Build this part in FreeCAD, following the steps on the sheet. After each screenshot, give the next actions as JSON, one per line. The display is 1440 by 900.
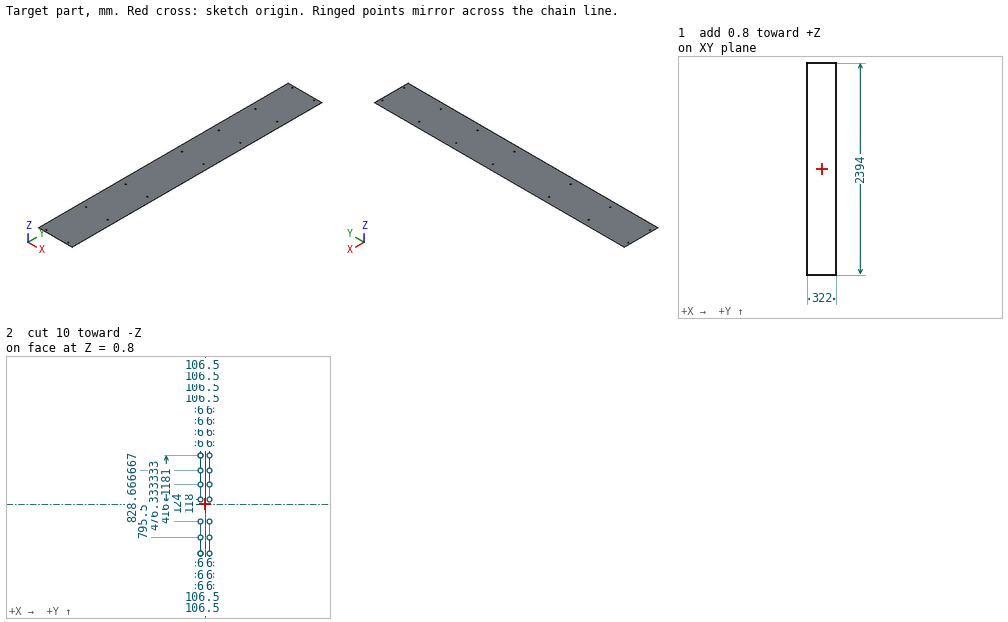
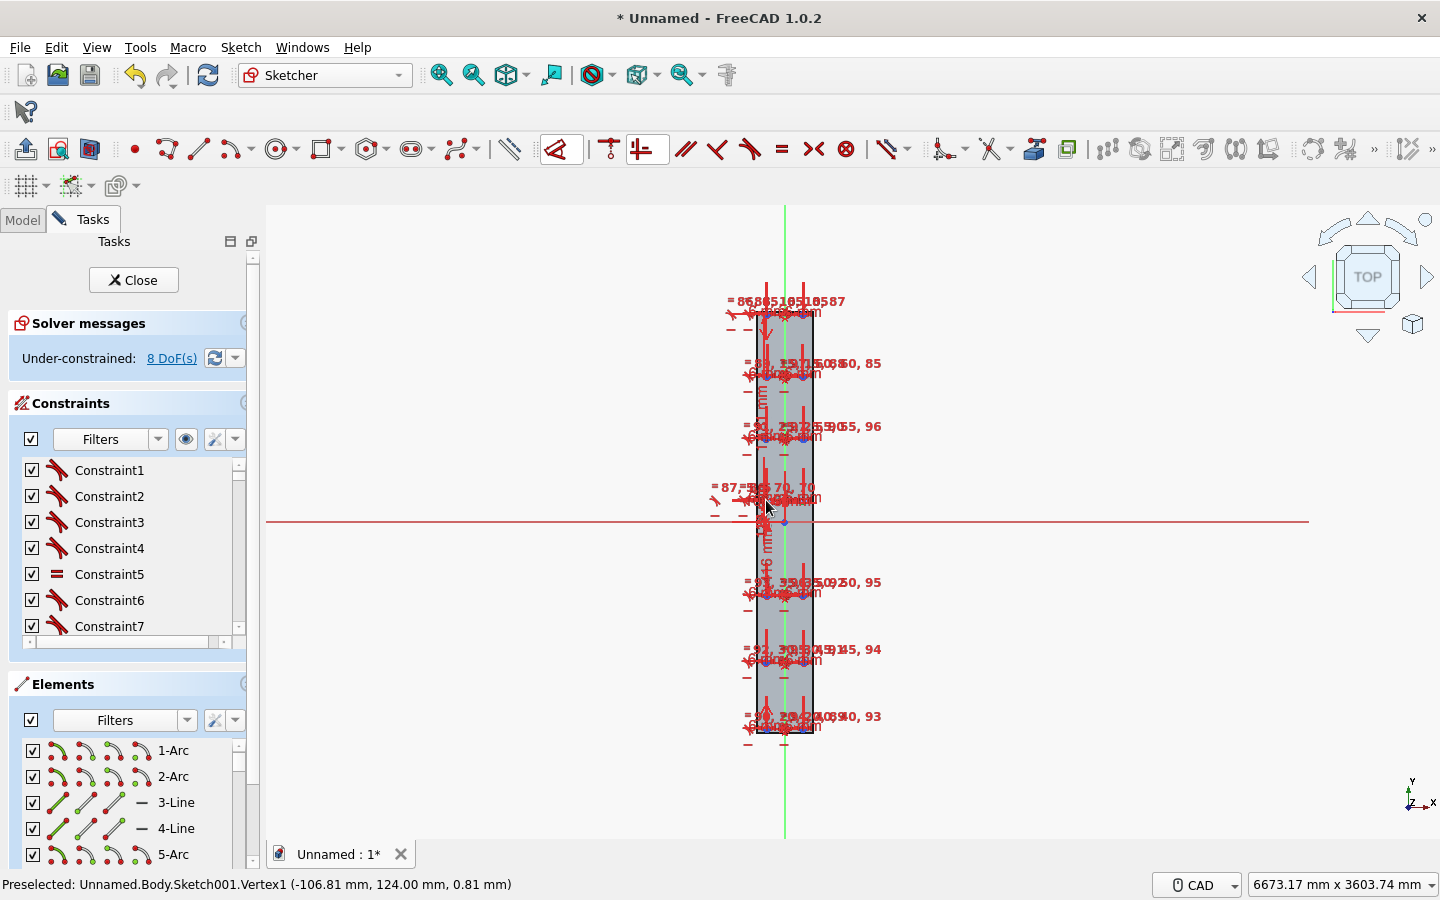
{"action": "scroll", "coordinate": [766, 314], "scroll_direction": "up", "scroll_amount": 14}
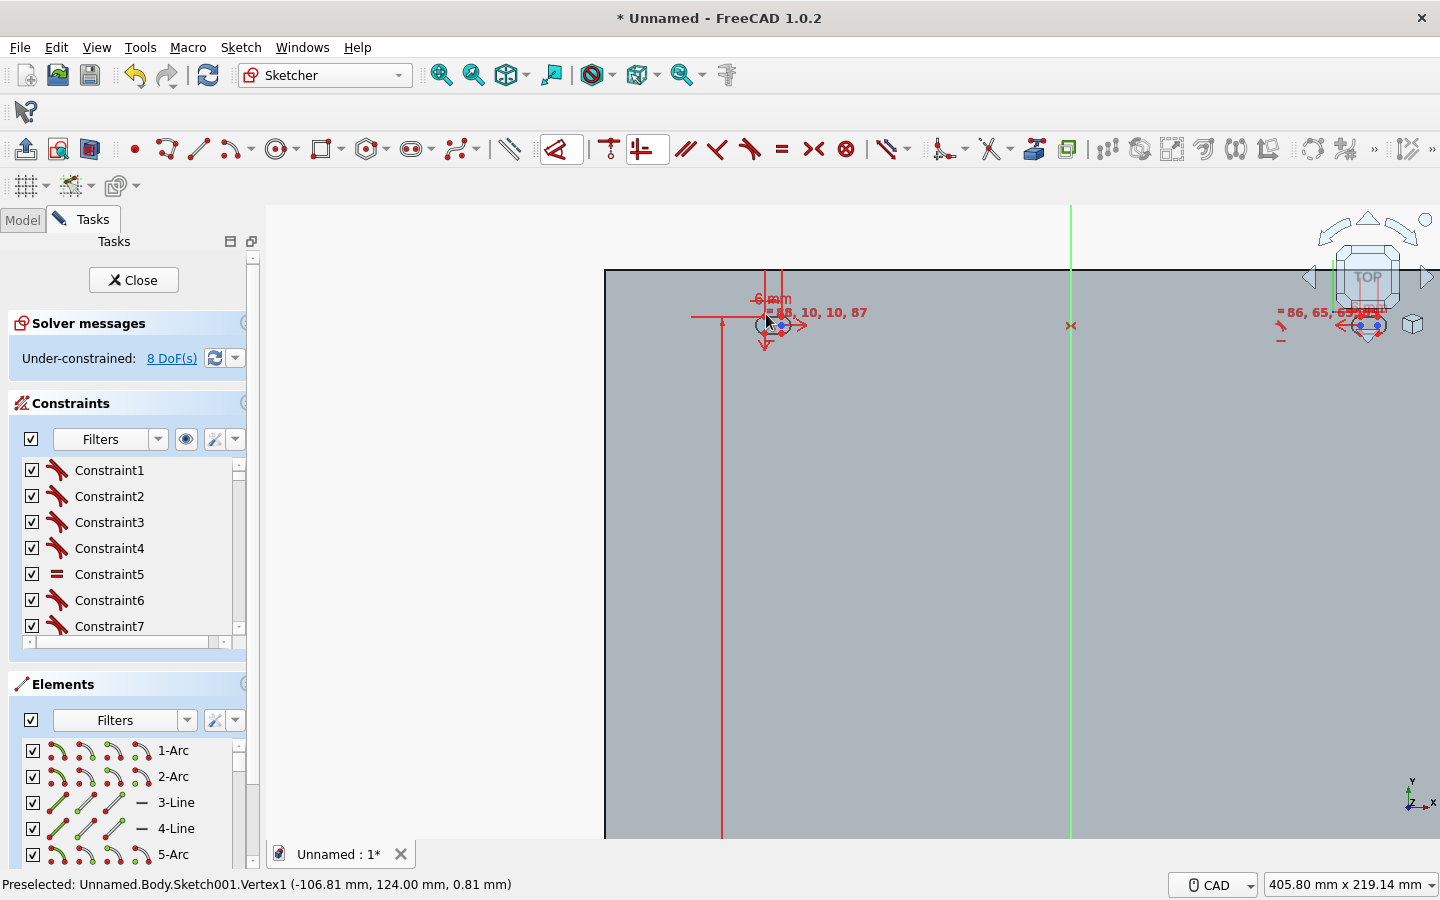
{"action": "left_click", "coordinate": [765, 317]}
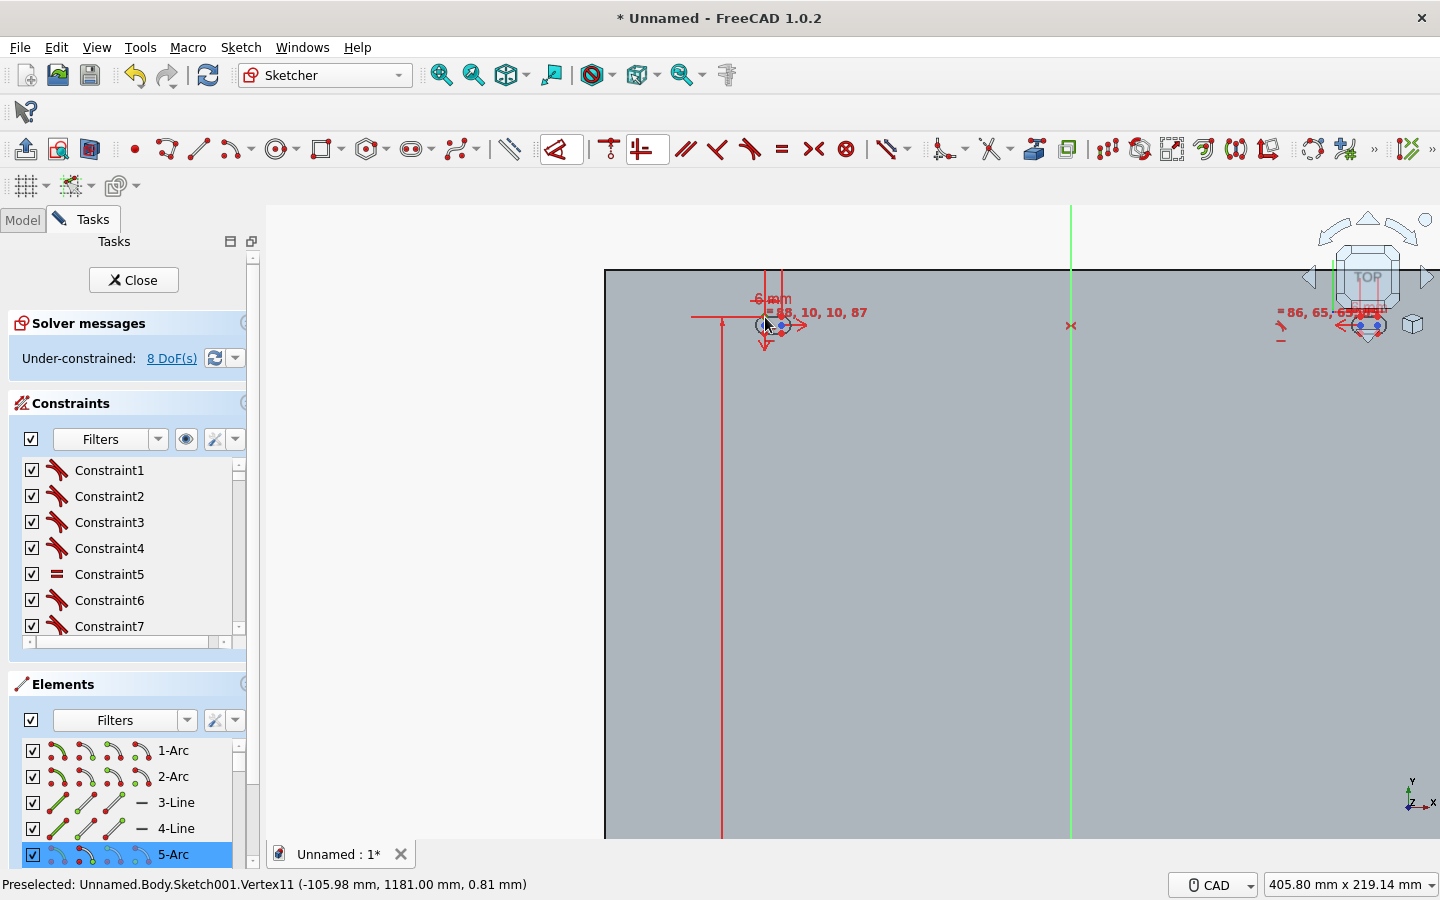
{"action": "key", "text": "l"}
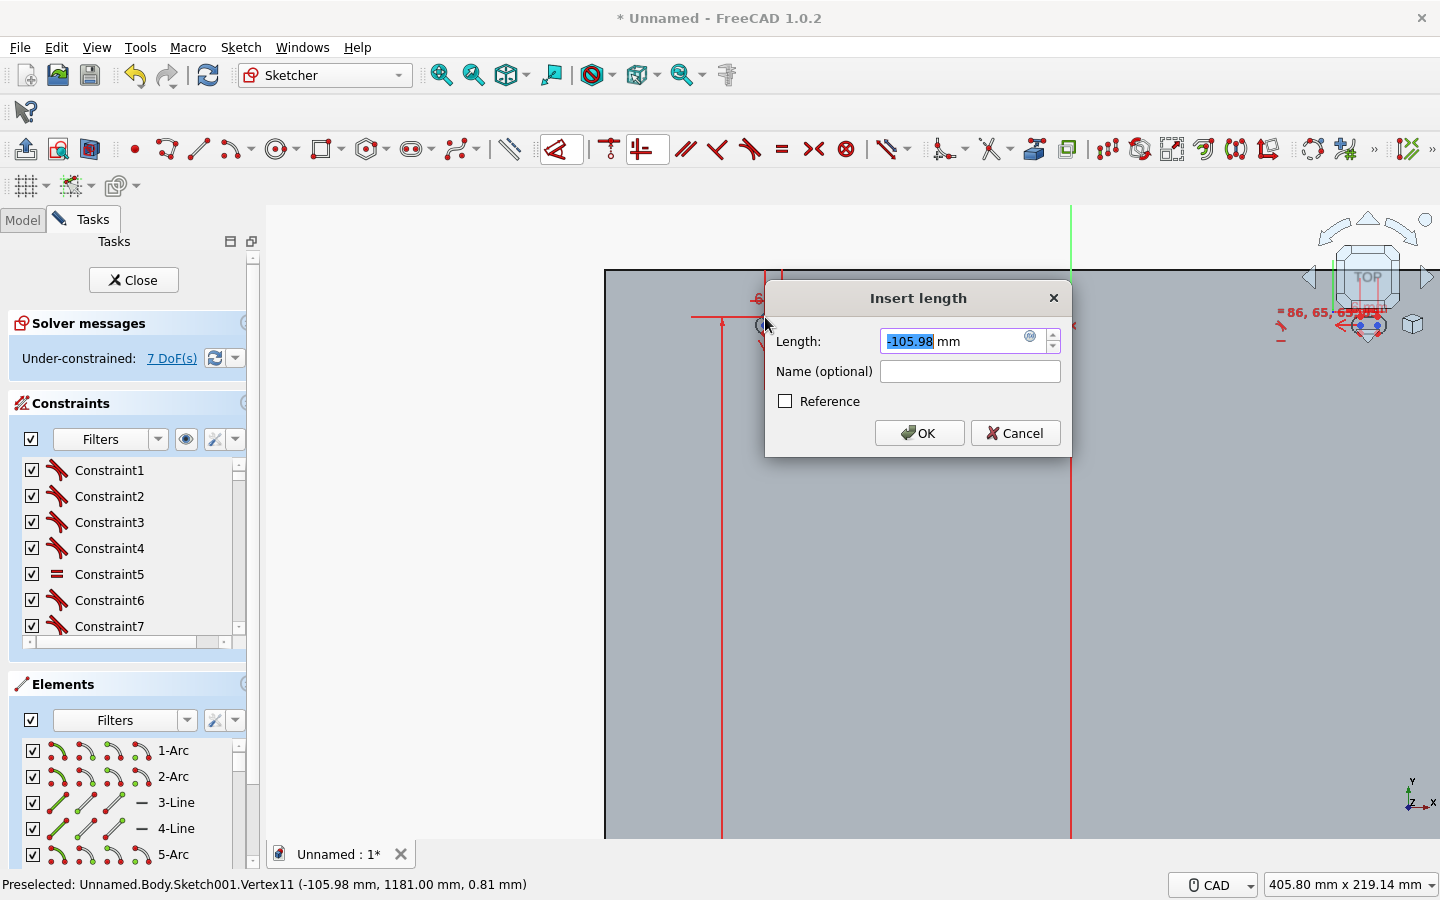
{"action": "type", "text": "-106.5"}
{"action": "key", "text": "Return"}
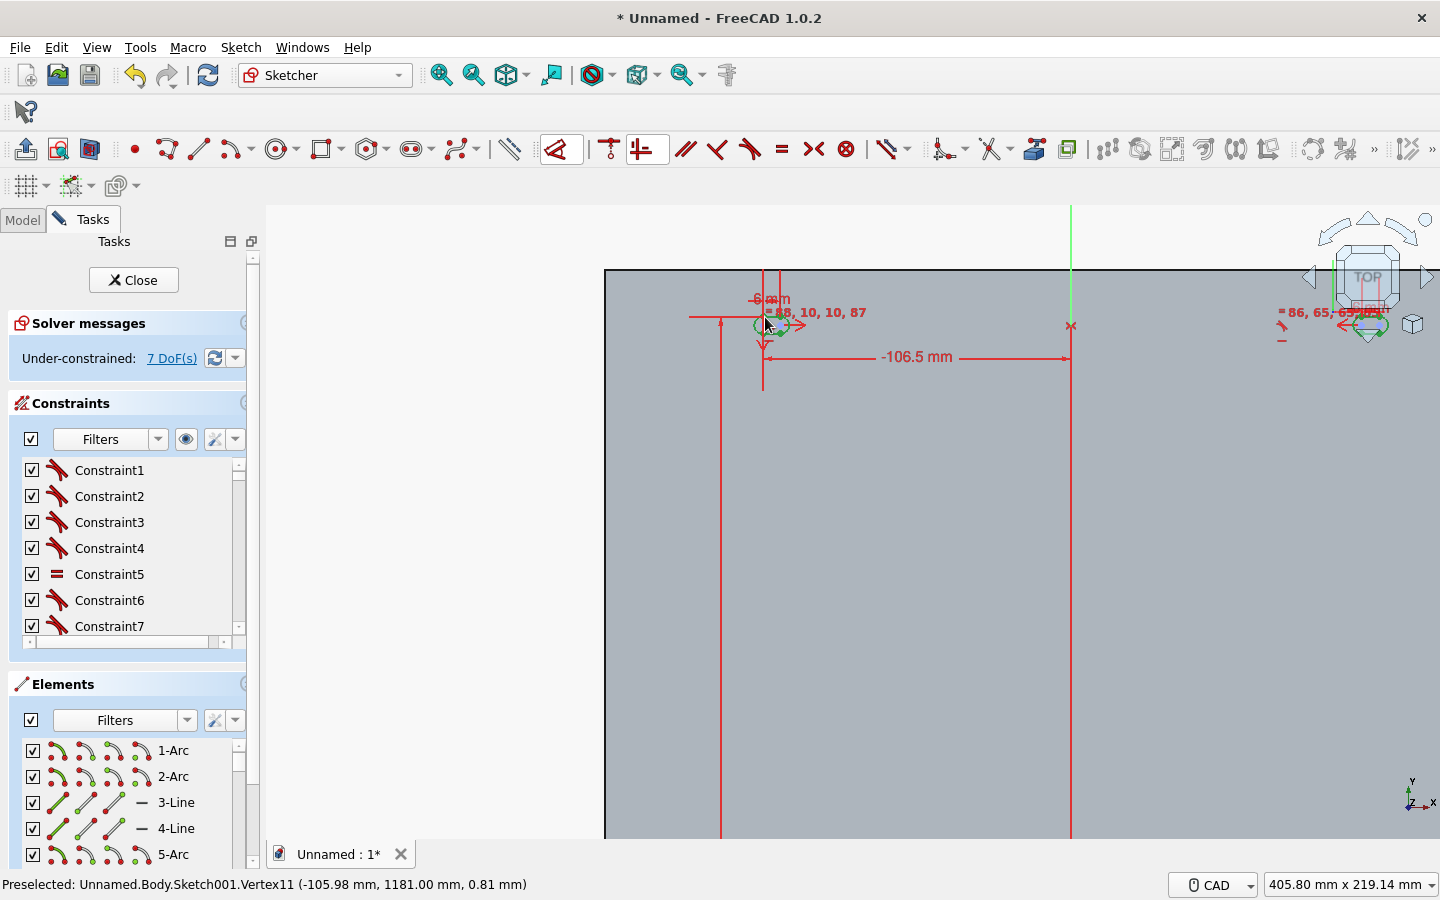
{"action": "scroll", "coordinate": [766, 314], "scroll_direction": "down", "scroll_amount": 14}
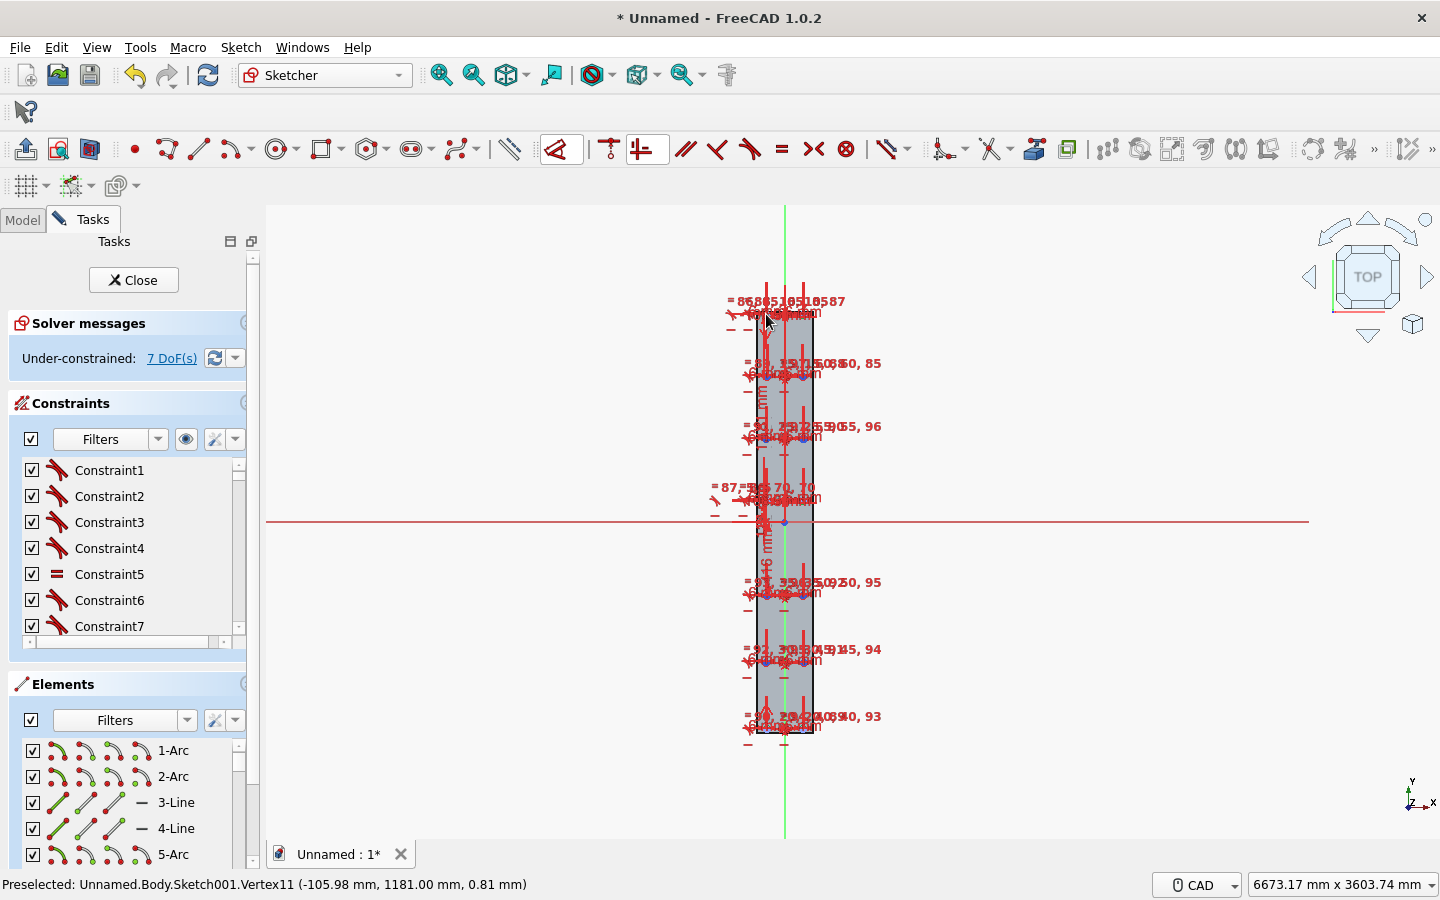
{"action": "scroll", "coordinate": [767, 376], "scroll_direction": "up", "scroll_amount": 14}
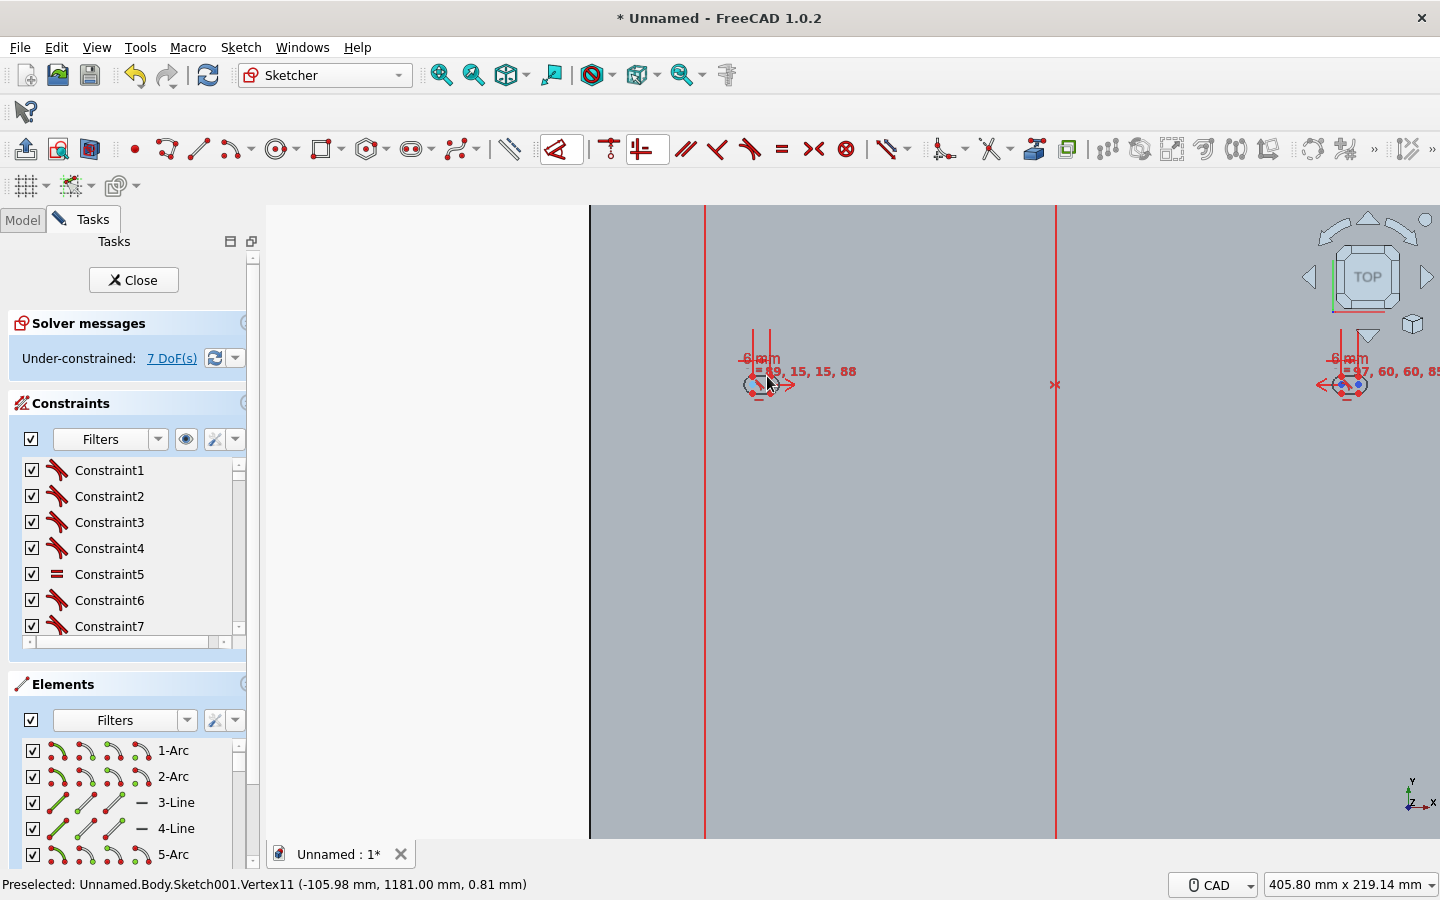
{"action": "left_click", "coordinate": [753, 376]}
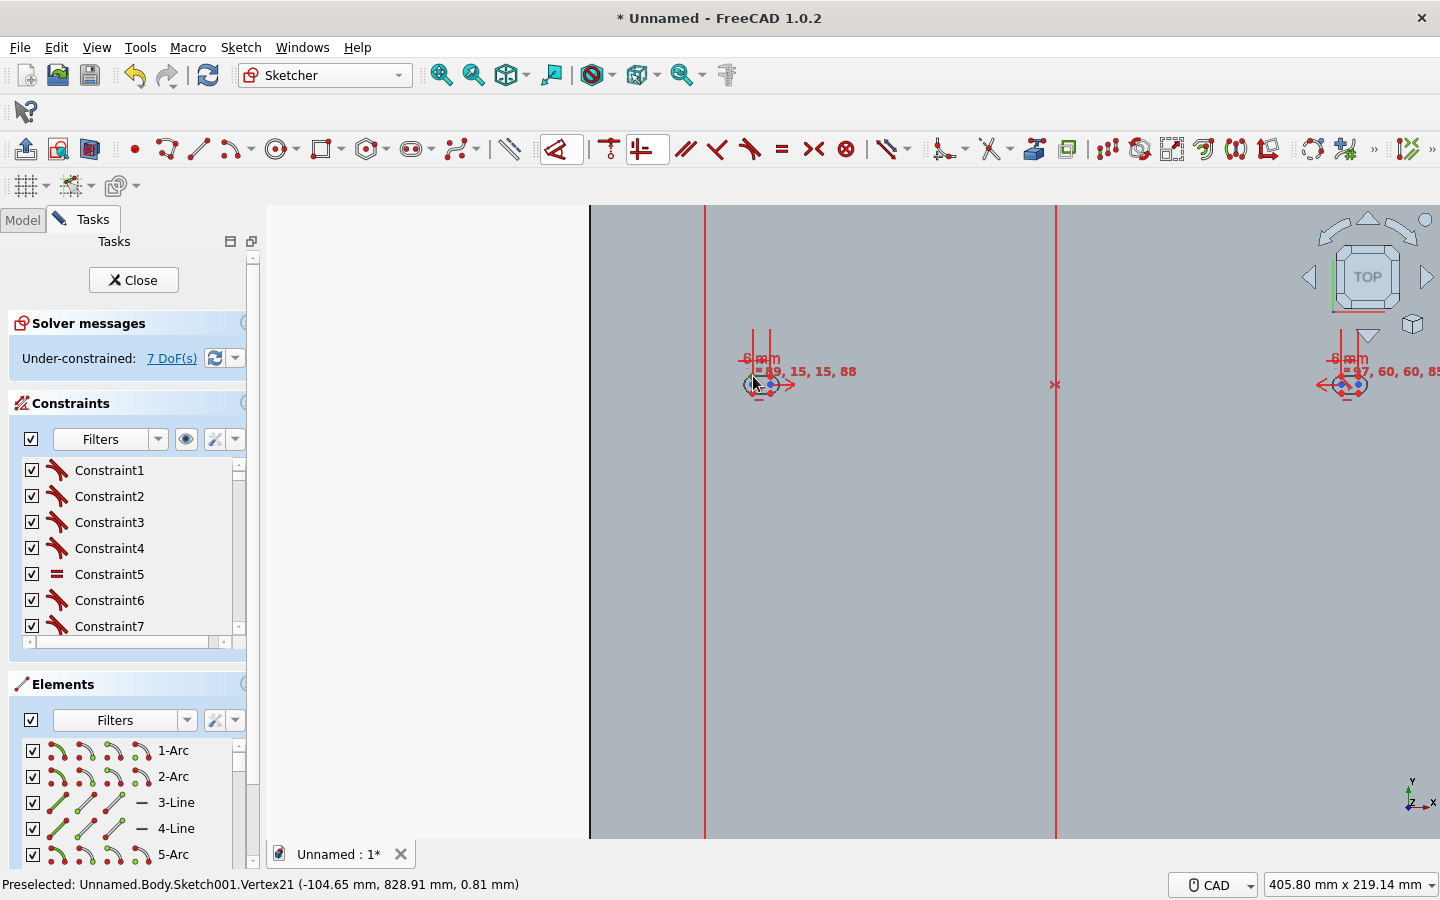
{"action": "key", "text": "l"}